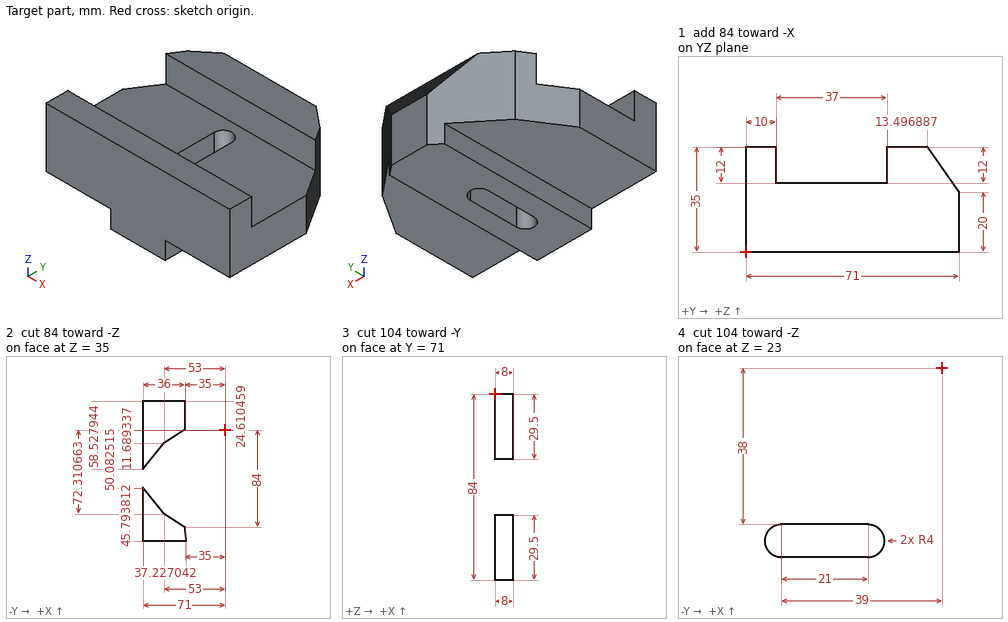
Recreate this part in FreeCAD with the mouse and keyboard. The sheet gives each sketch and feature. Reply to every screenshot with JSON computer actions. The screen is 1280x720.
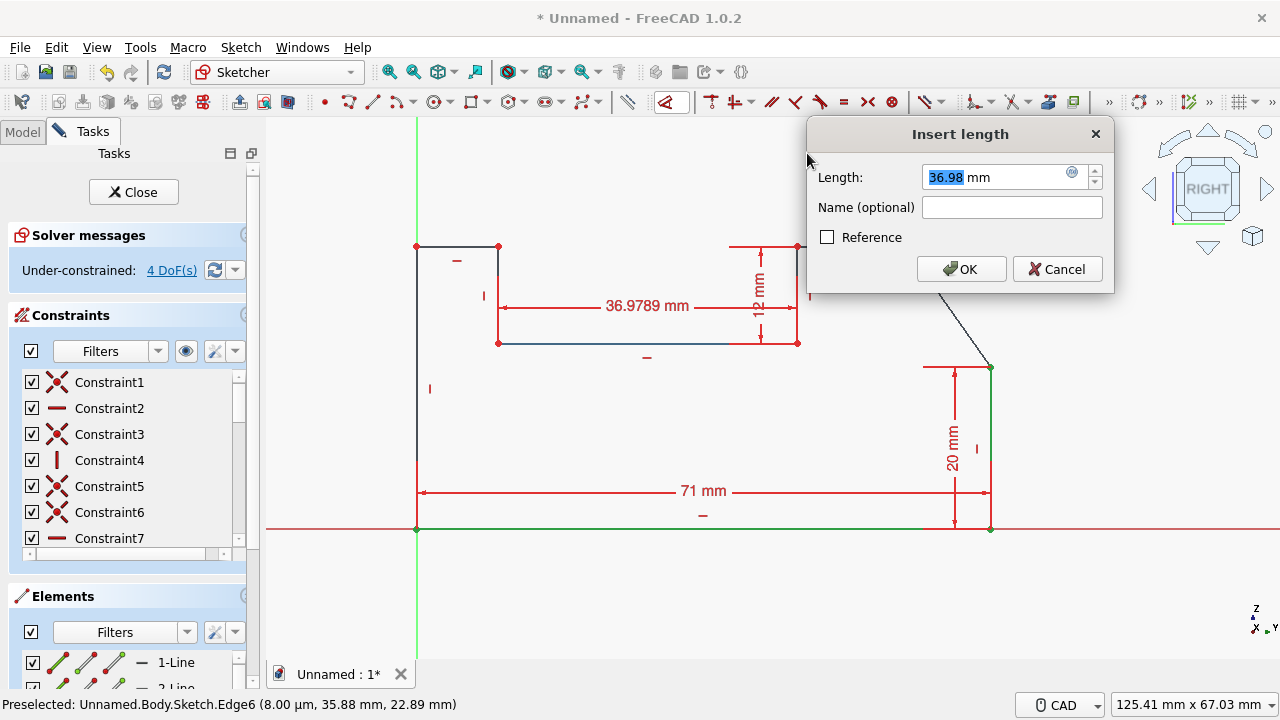
{"action": "type", "text": "37"}
{"action": "key", "text": "Return"}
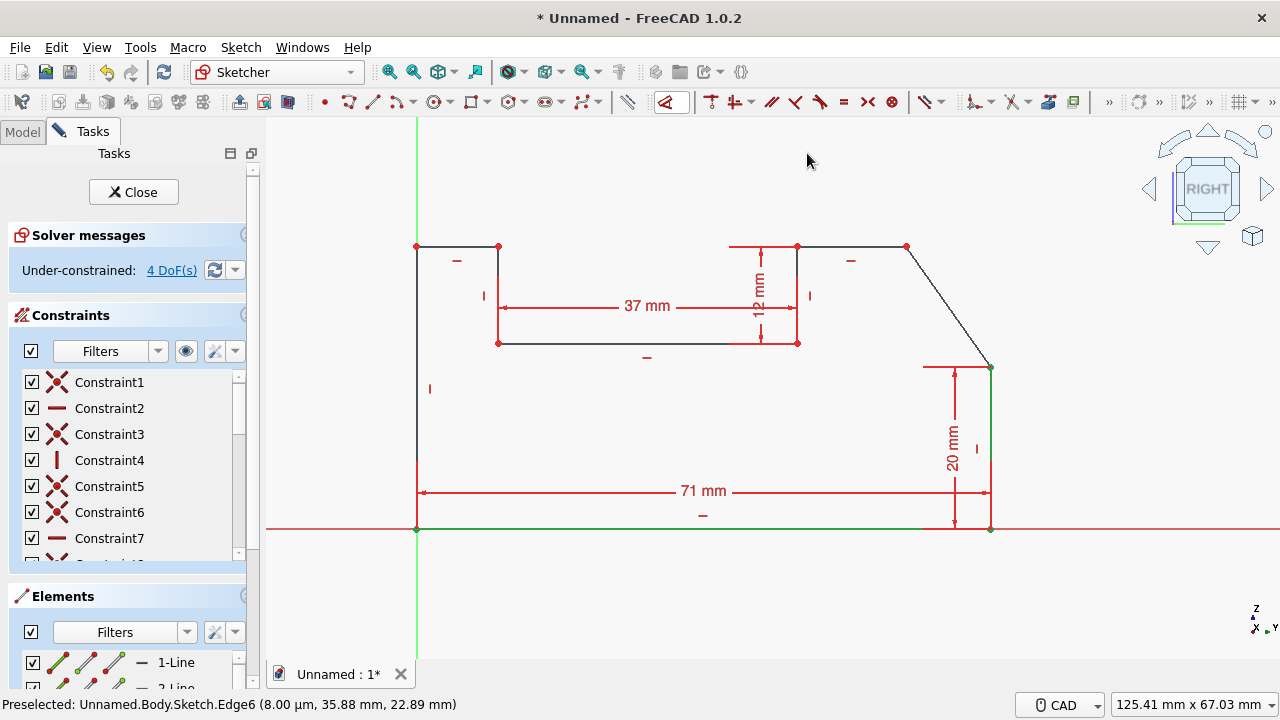
{"action": "left_click", "coordinate": [498, 315]}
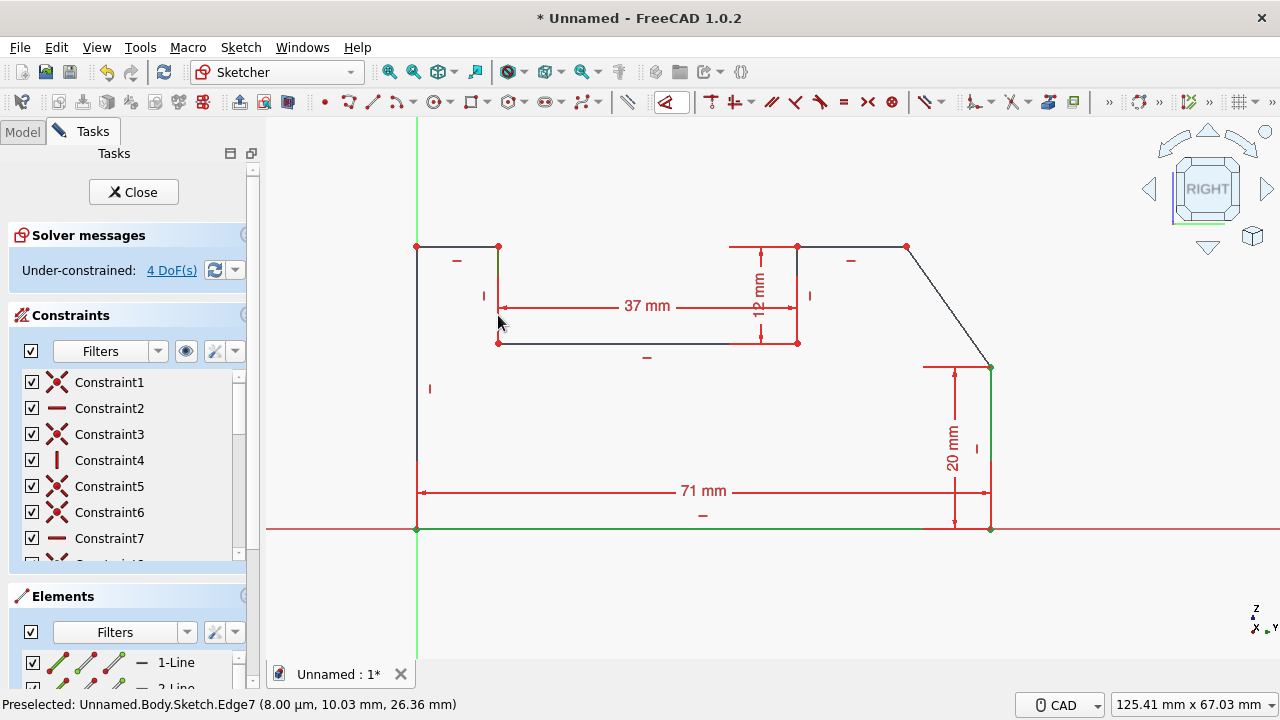
{"action": "left_click", "coordinate": [684, 102]}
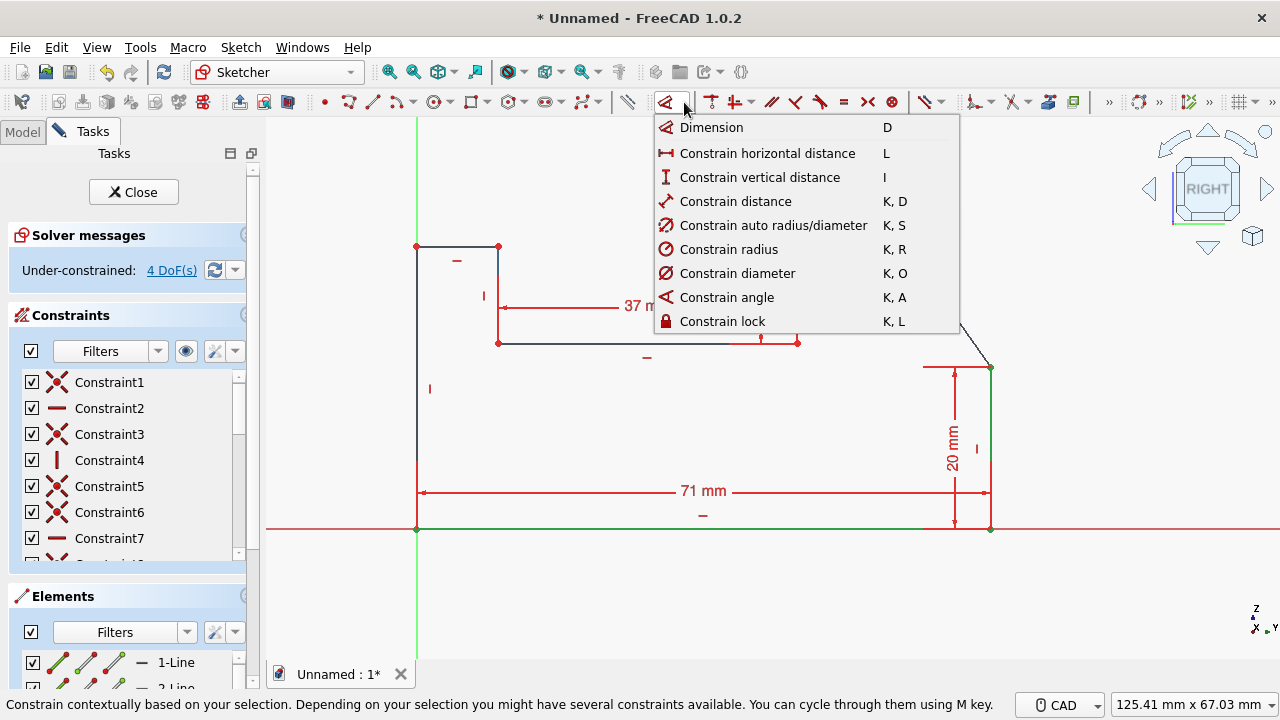
{"action": "left_click", "coordinate": [807, 177]}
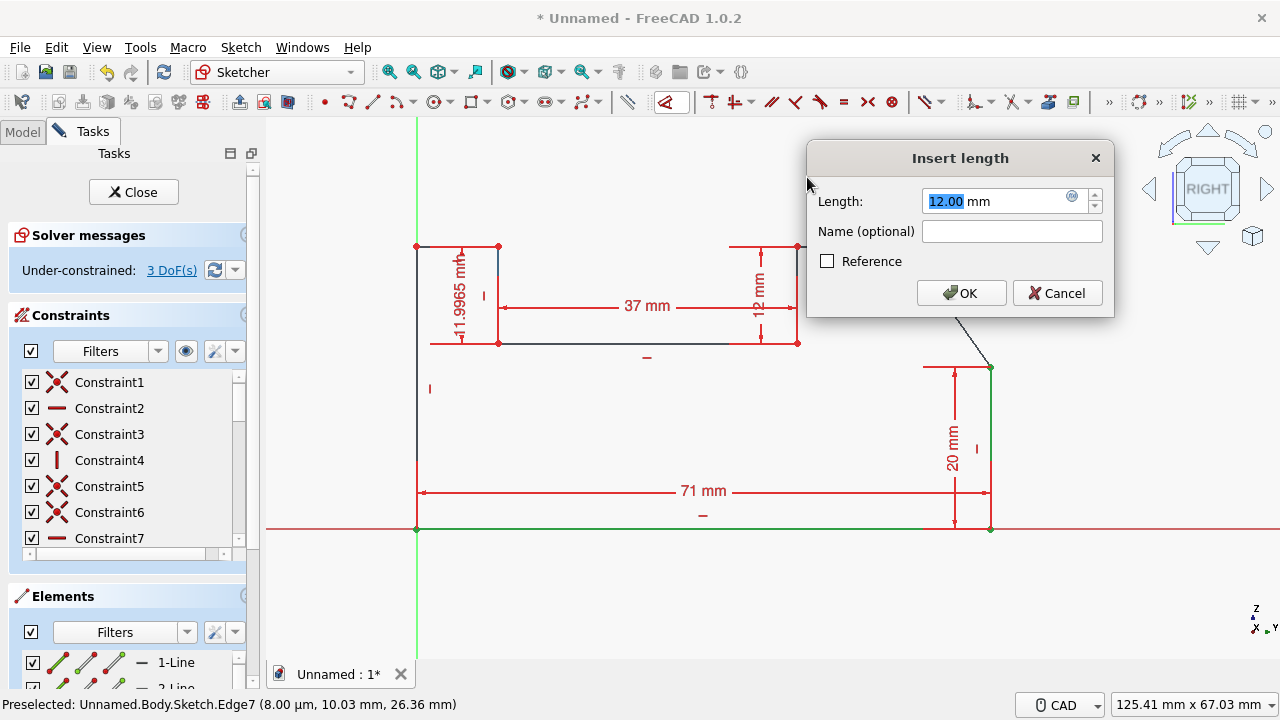
{"action": "type", "text": "12"}
{"action": "key", "text": "Return"}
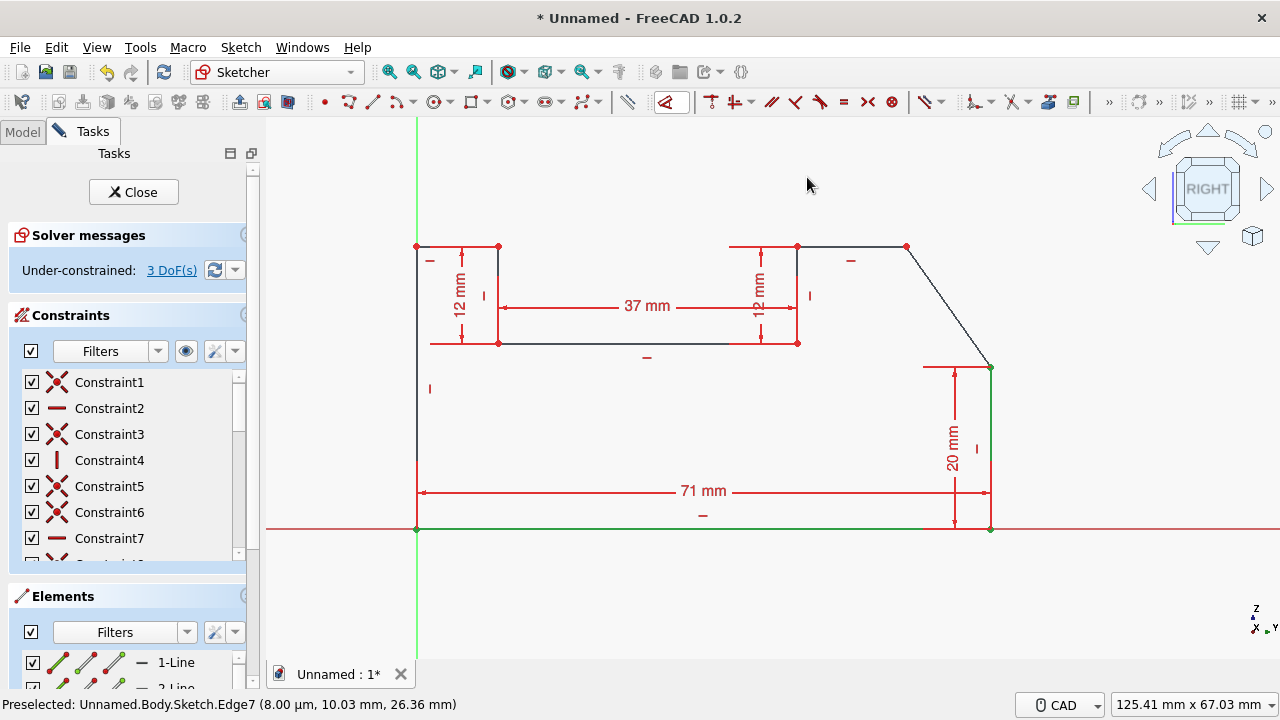
{"action": "left_click", "coordinate": [474, 247]}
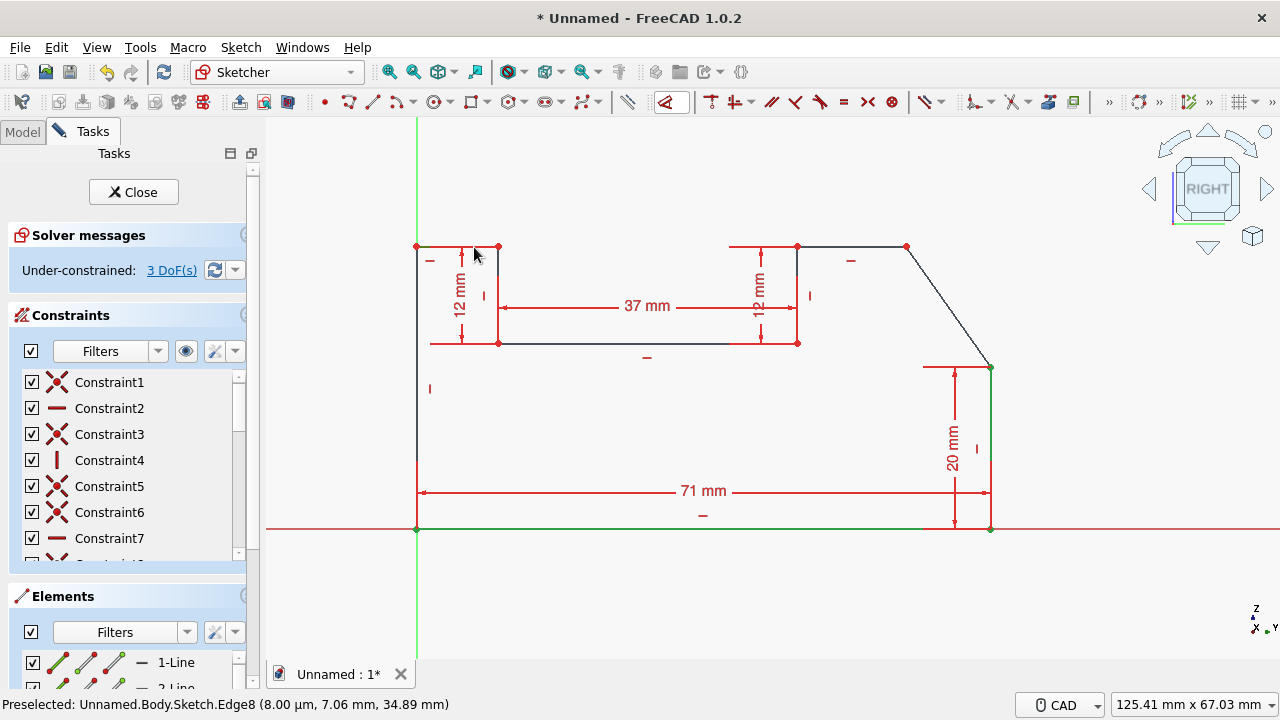
{"action": "left_click", "coordinate": [684, 102]}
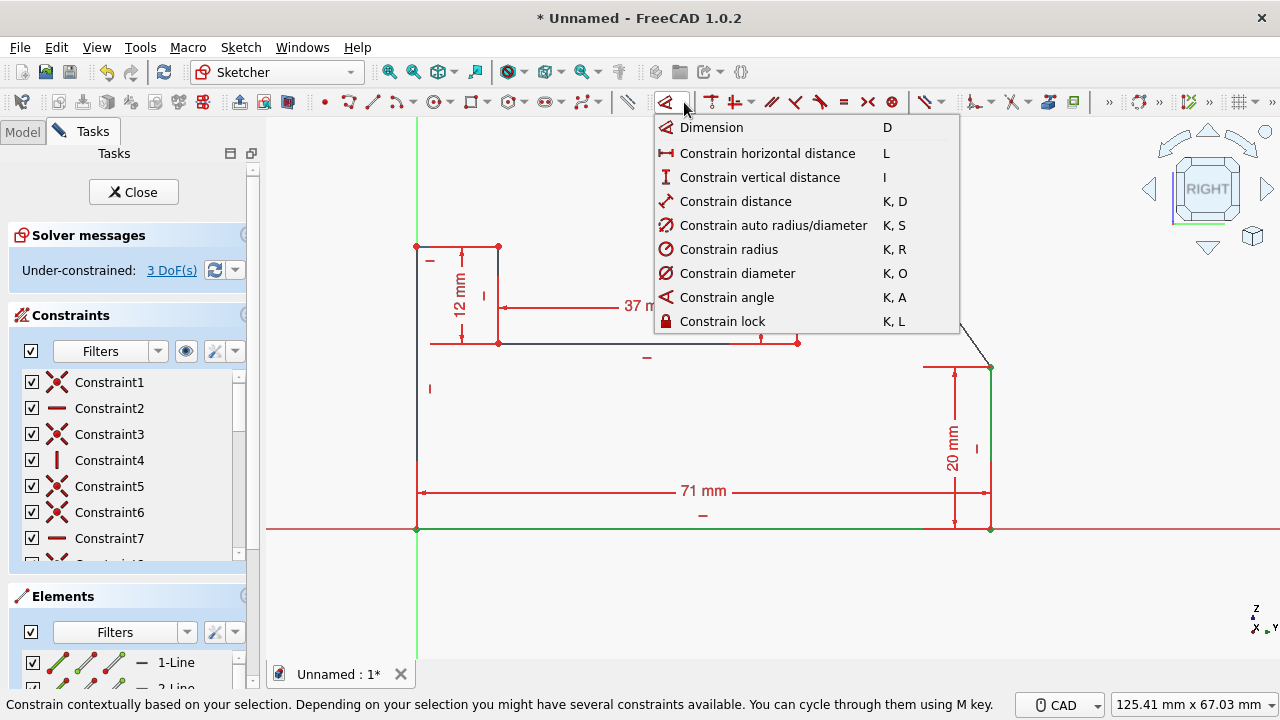
{"action": "left_click", "coordinate": [807, 153]}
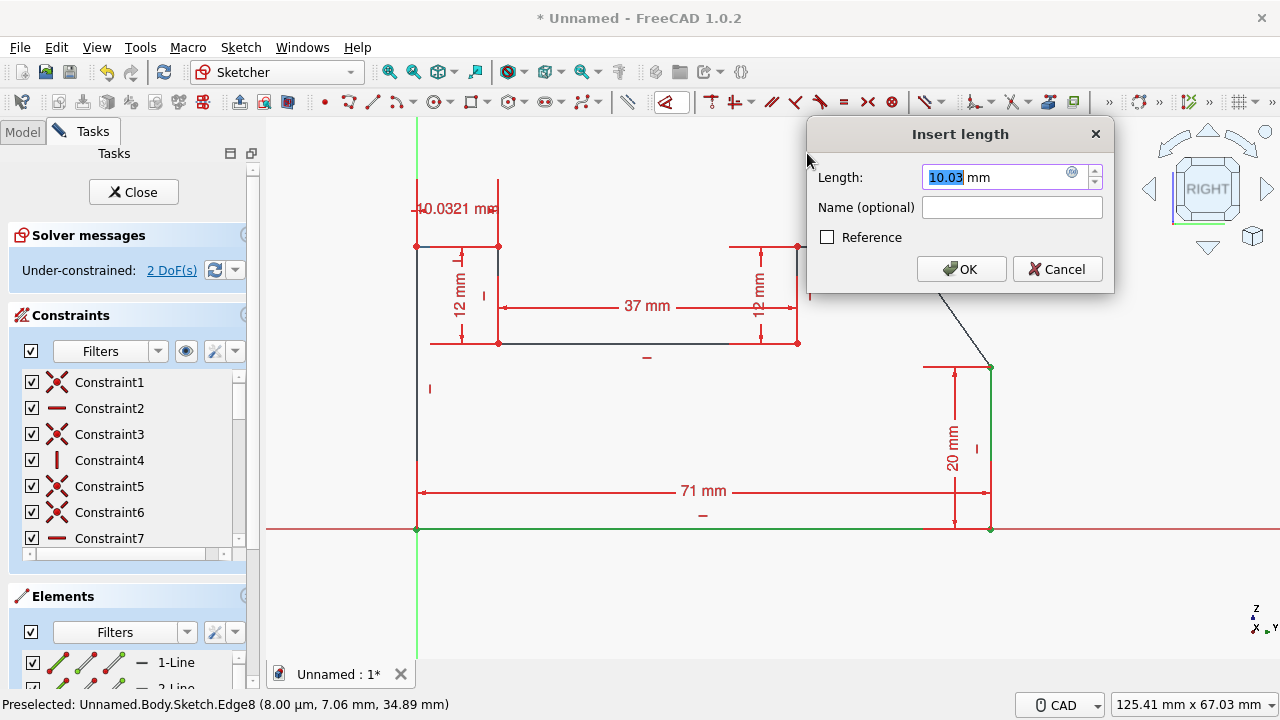
{"action": "type", "text": "10"}
{"action": "key", "text": "Return"}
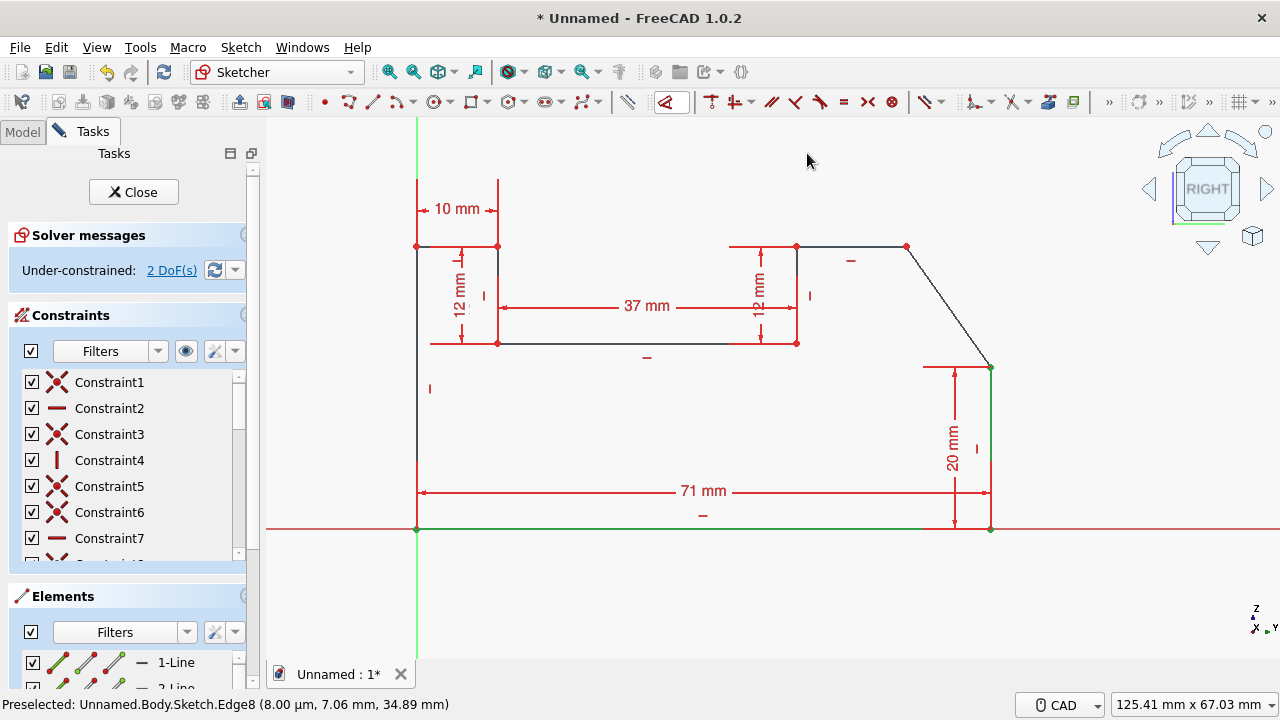
{"action": "left_click", "coordinate": [417, 332]}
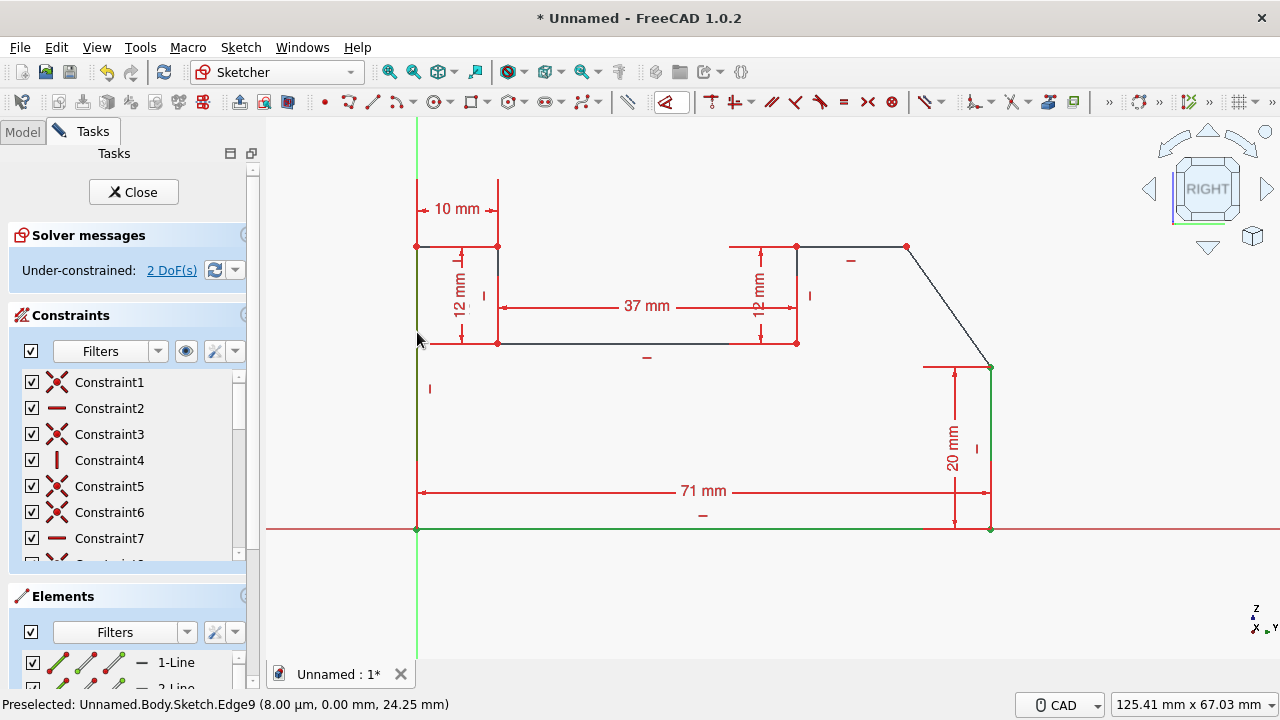
{"action": "left_click", "coordinate": [684, 102]}